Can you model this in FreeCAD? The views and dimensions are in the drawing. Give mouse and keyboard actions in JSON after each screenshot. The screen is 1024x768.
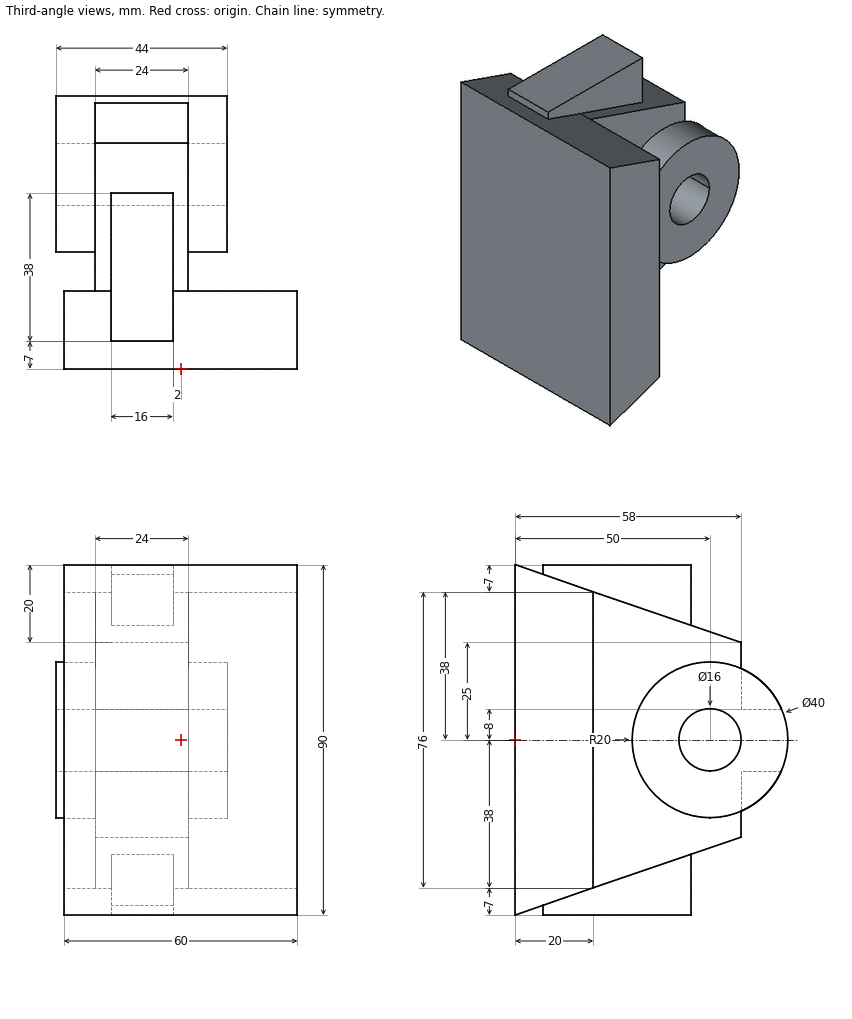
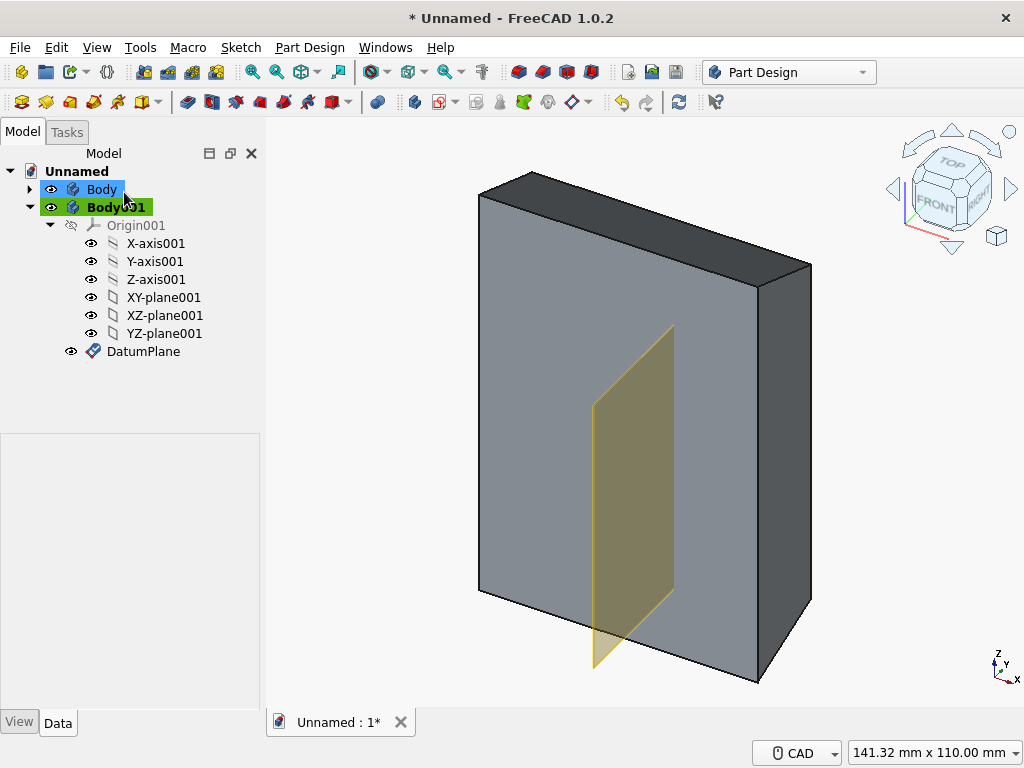
{"action": "left_click", "coordinate": [116, 351]}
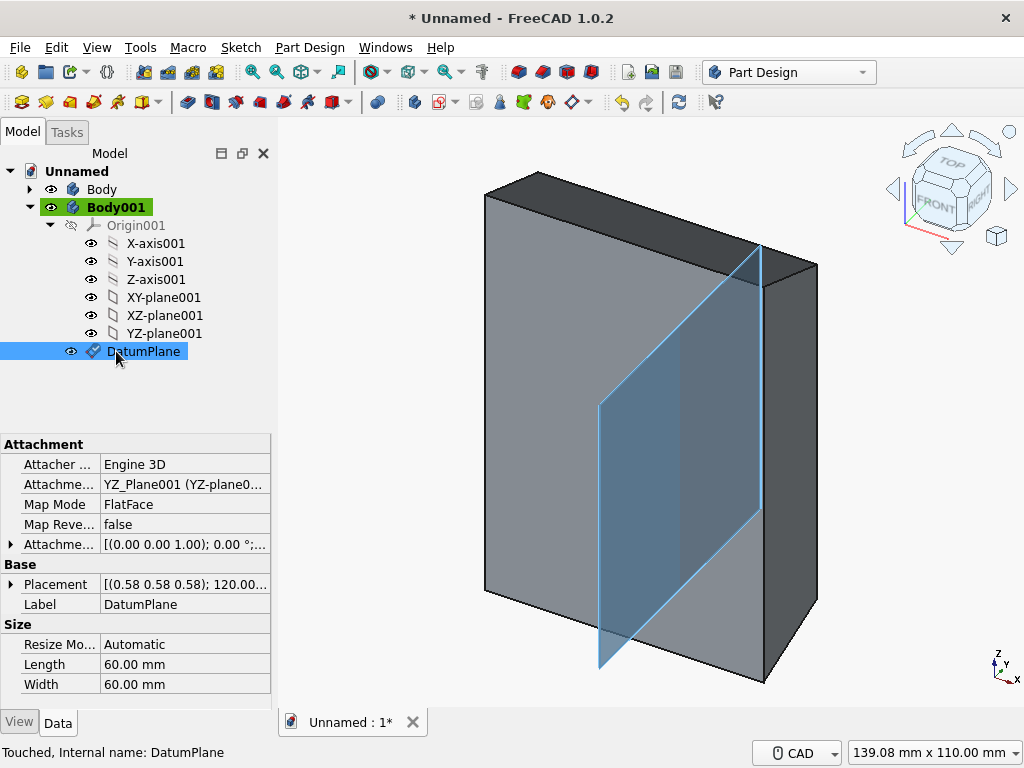
{"action": "left_click", "coordinate": [440, 102]}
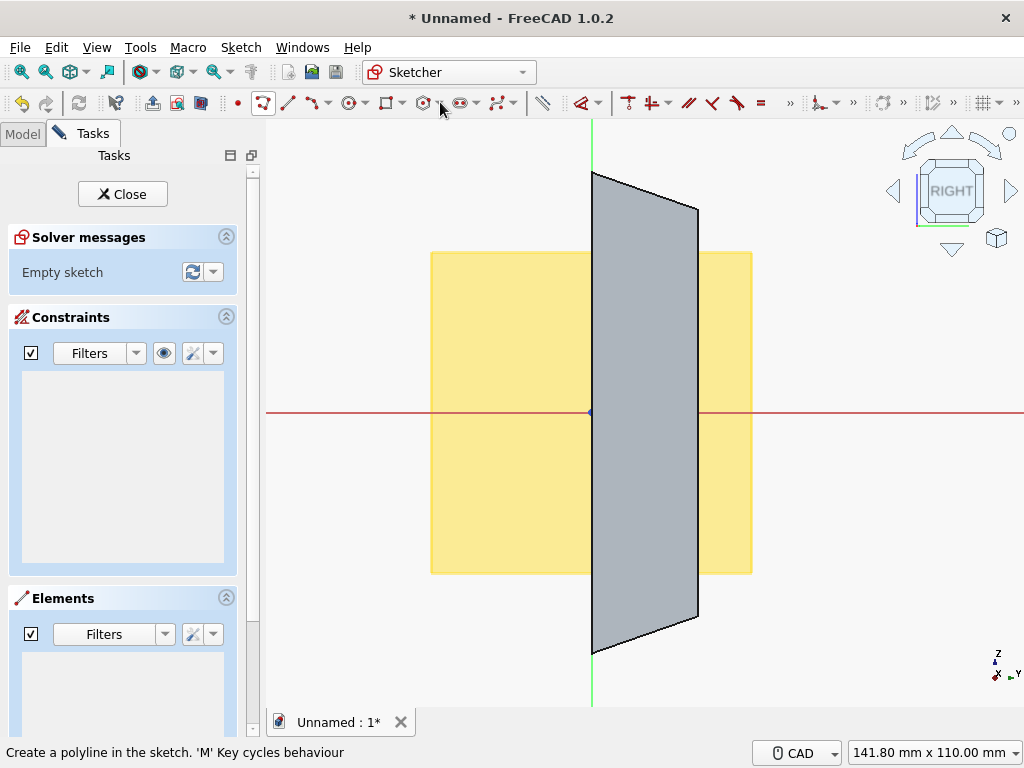
{"action": "scroll", "coordinate": [294, 413], "scroll_direction": "down", "scroll_amount": 2}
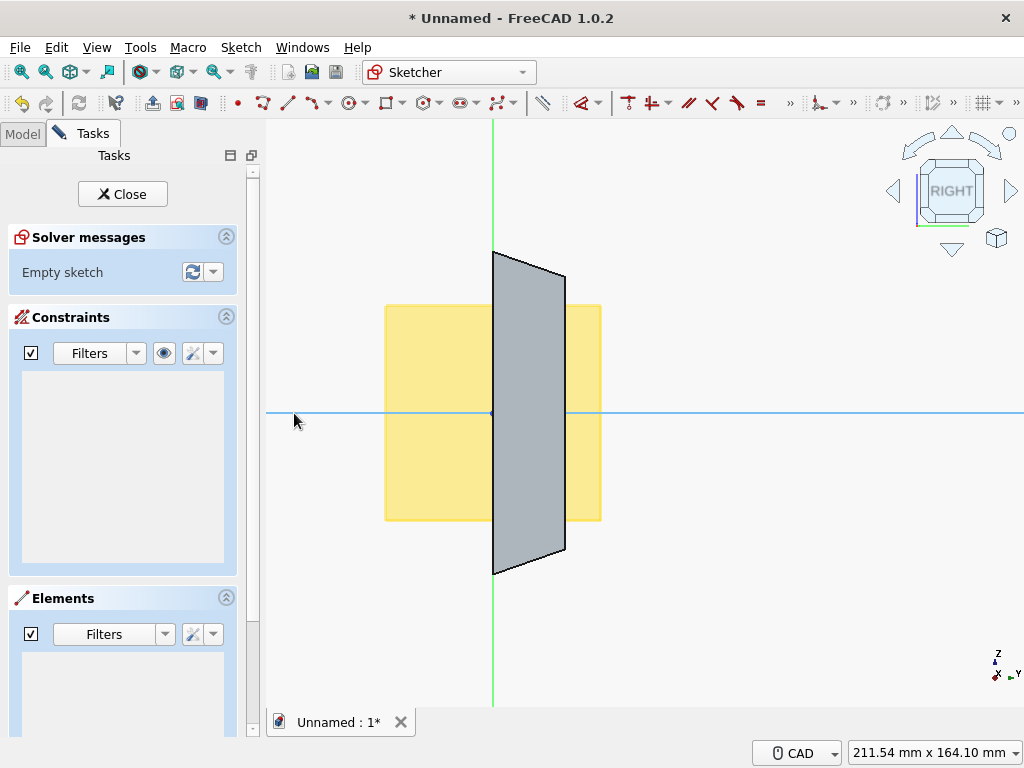
{"action": "scroll", "coordinate": [705, 414], "scroll_direction": "up", "scroll_amount": 2}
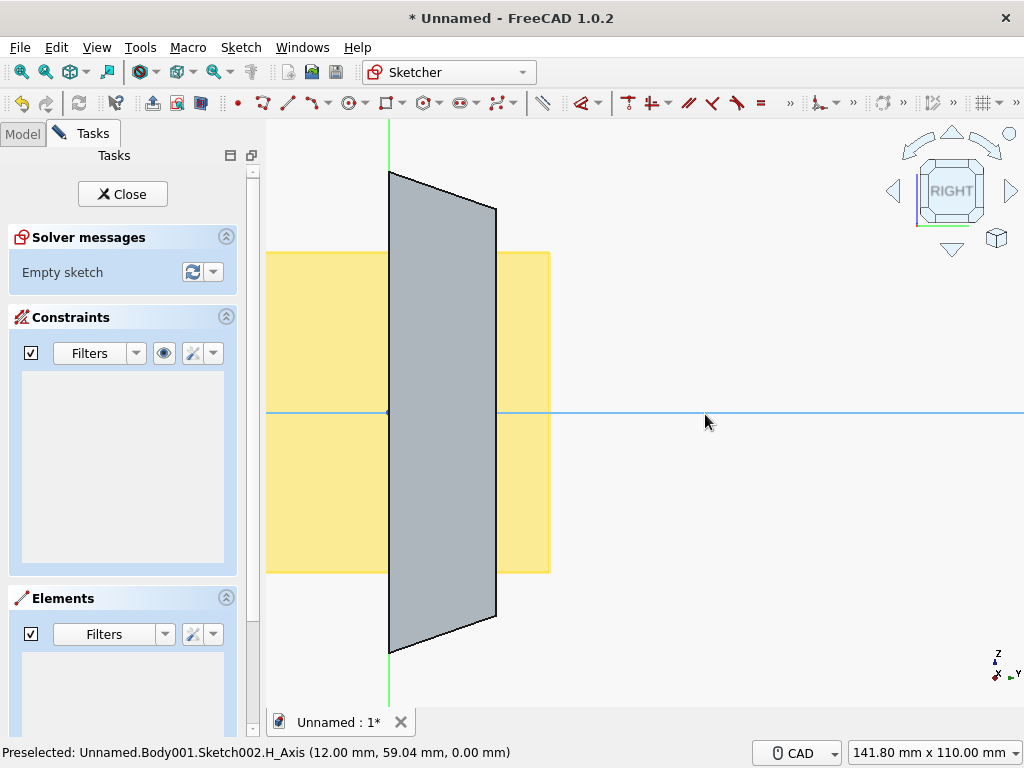
{"action": "left_click", "coordinate": [350, 104]}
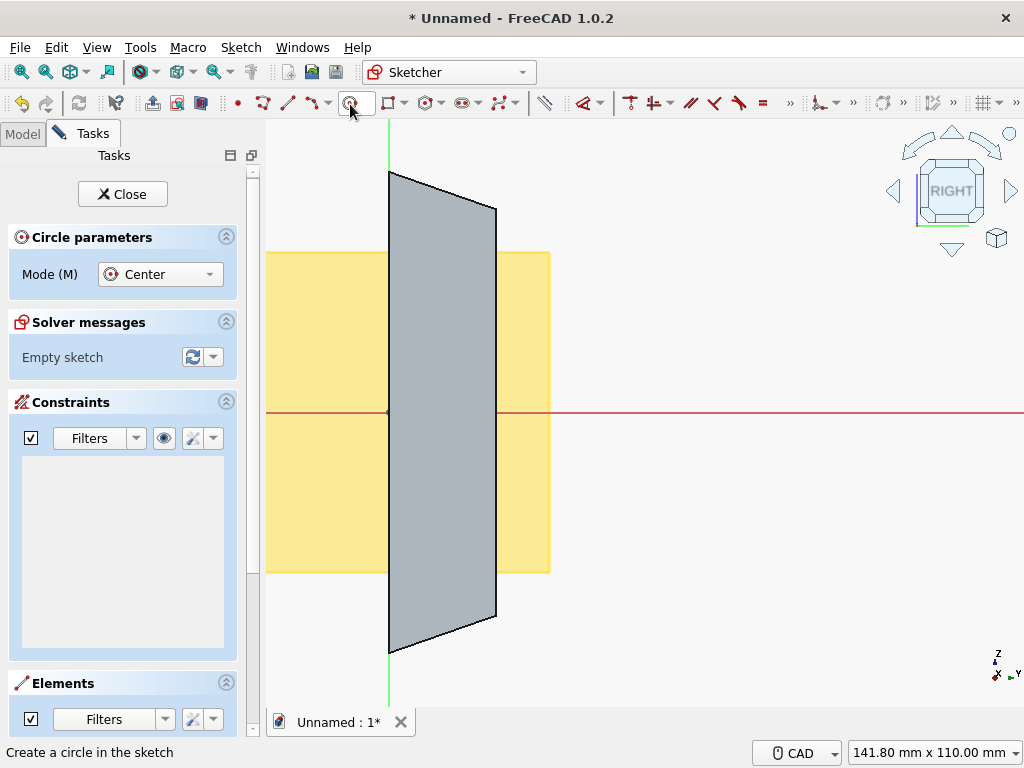
{"action": "left_click", "coordinate": [656, 413]}
{"action": "mouse_move", "coordinate": [732, 337]}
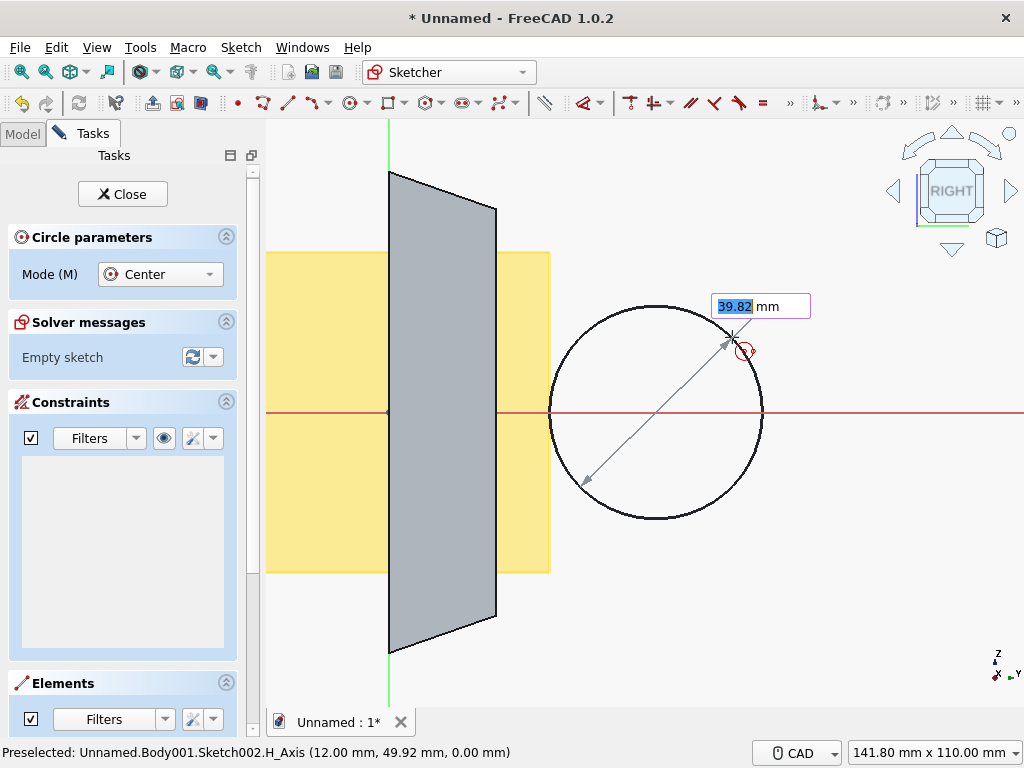
{"action": "type", "text": "40"}
{"action": "key", "text": "Return"}
{"action": "key", "text": "Escape"}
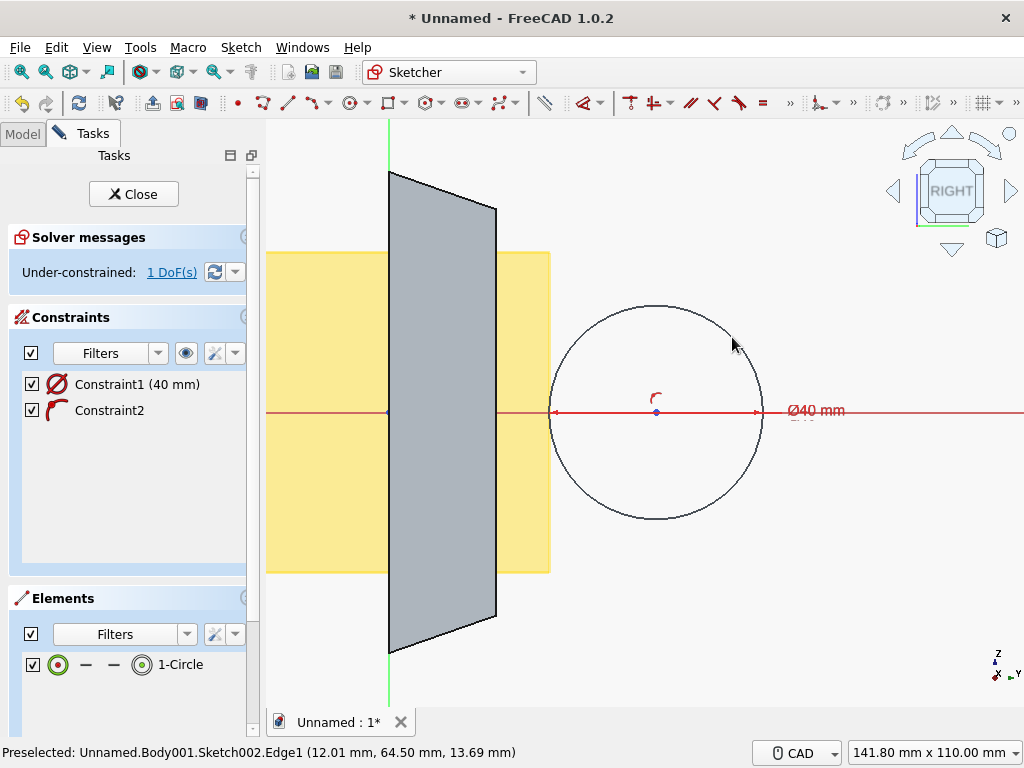
{"action": "key", "text": "d"}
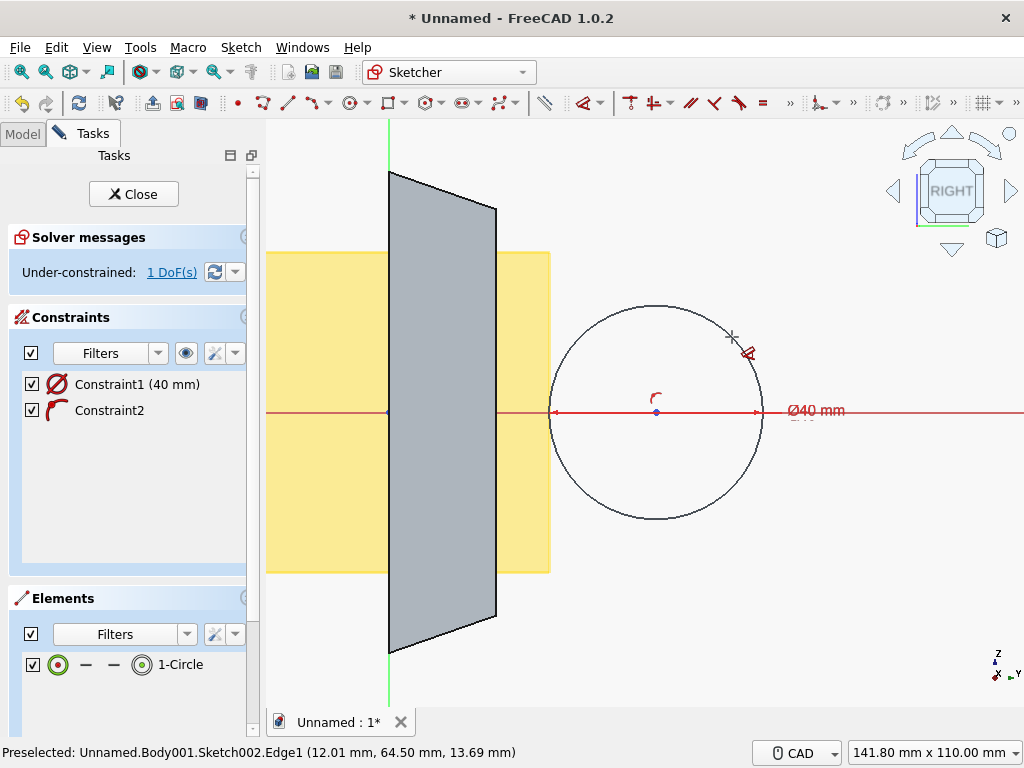
{"action": "left_click", "coordinate": [656, 413]}
{"action": "left_click", "coordinate": [523, 447]}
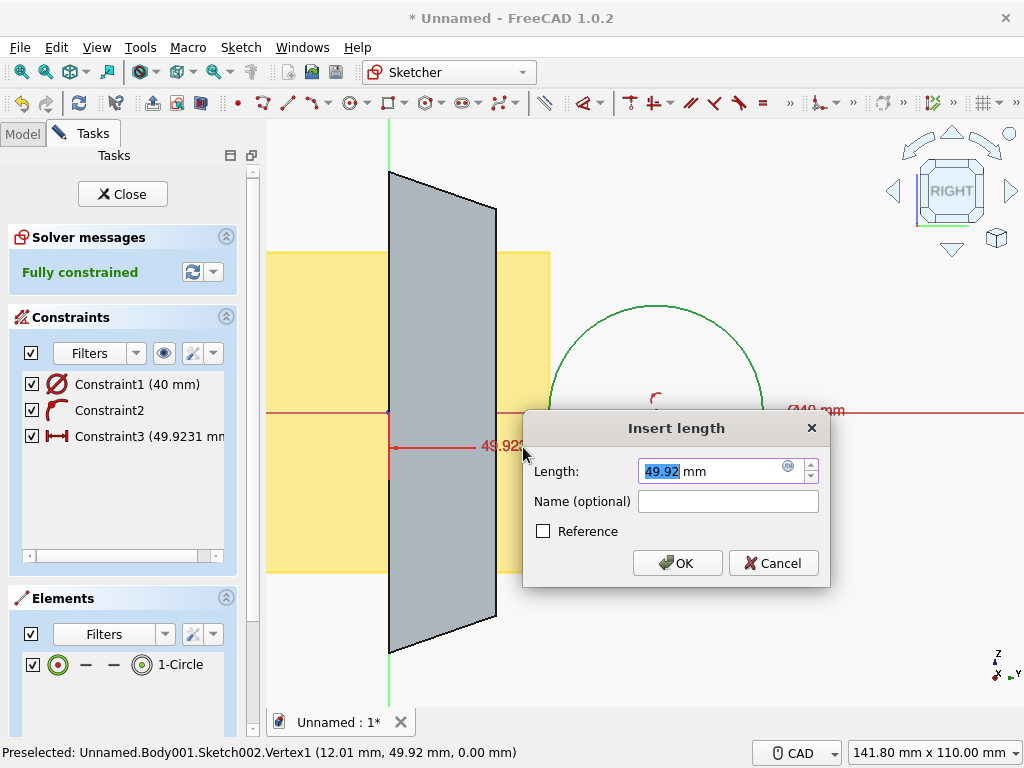
{"action": "type", "text": "50"}
{"action": "key", "text": "Return"}
{"action": "key", "text": "Escape"}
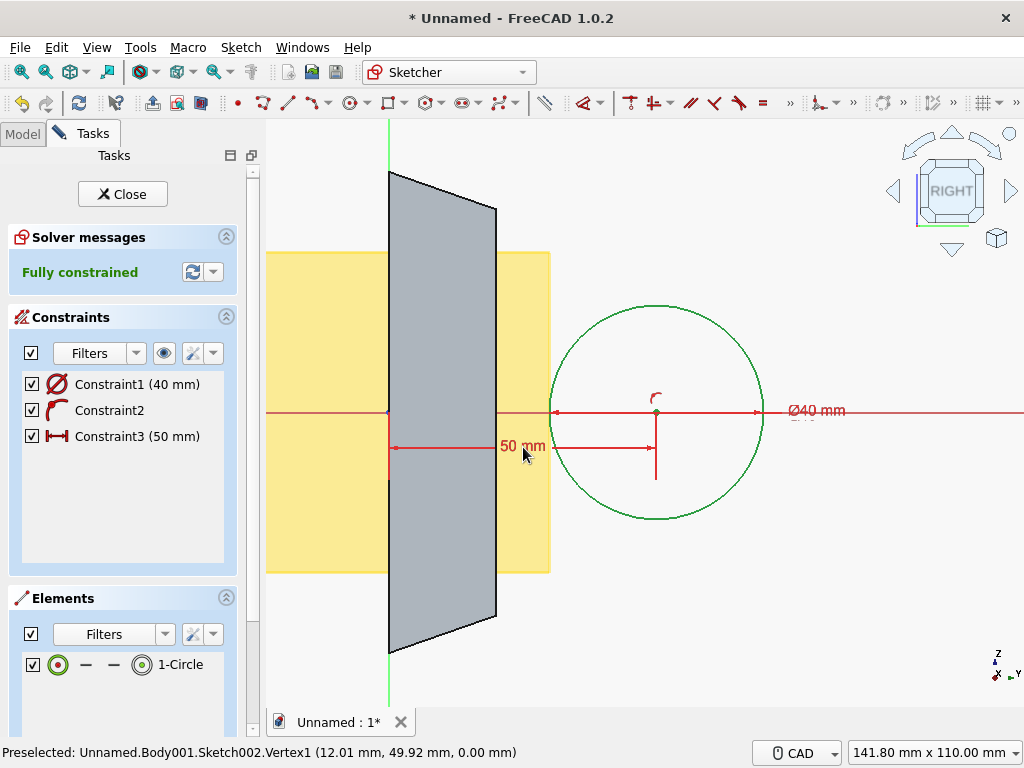
{"action": "left_click", "coordinate": [123, 194]}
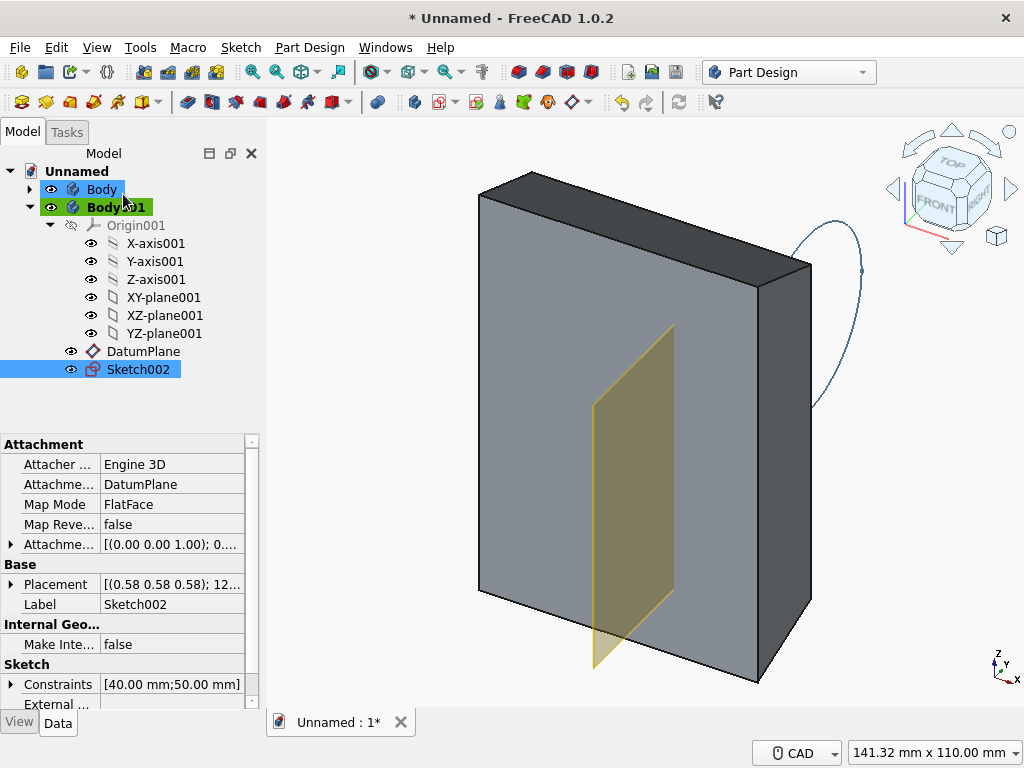
{"action": "left_click", "coordinate": [22, 102]}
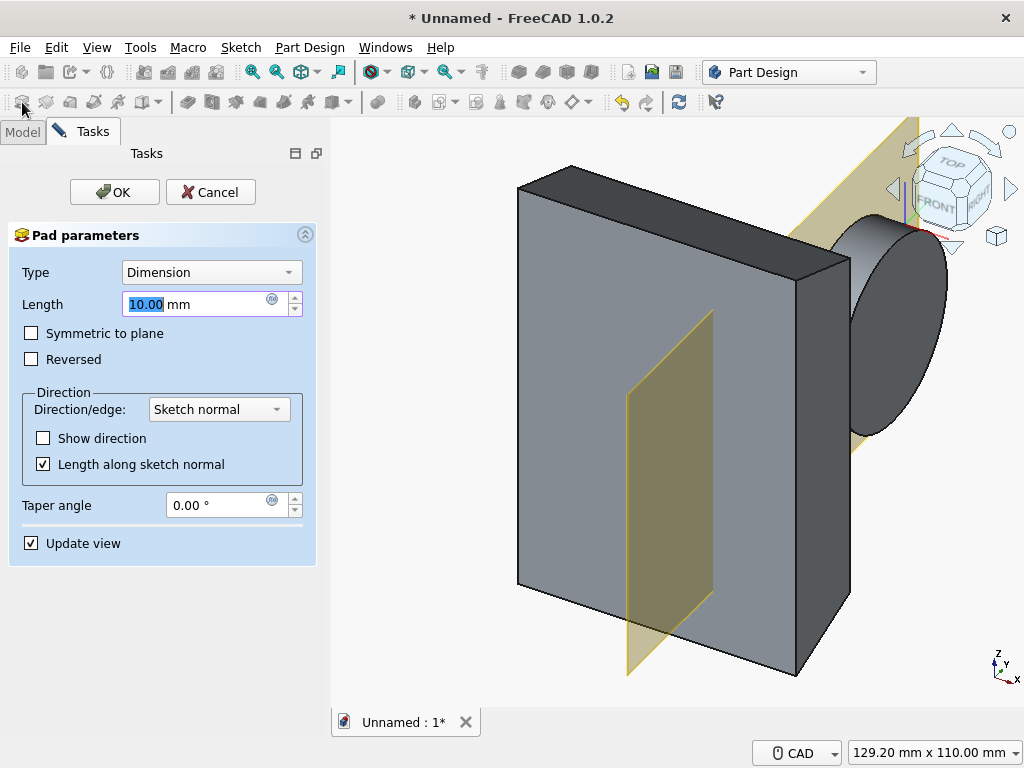
{"action": "type", "text": "44"}
{"action": "key", "text": "Tab"}